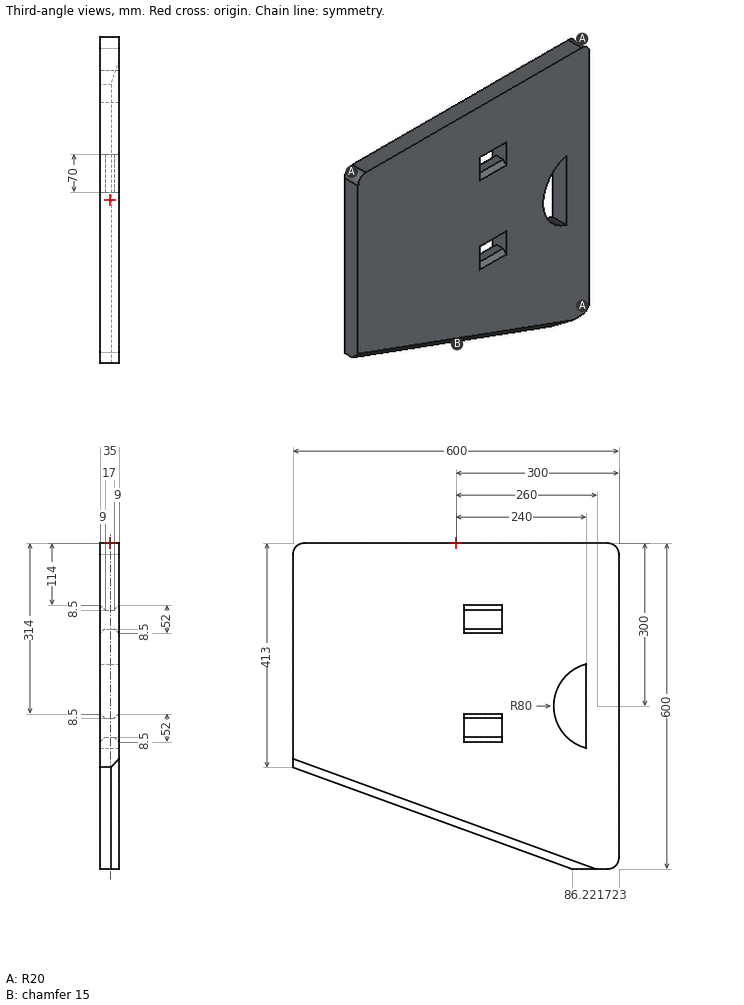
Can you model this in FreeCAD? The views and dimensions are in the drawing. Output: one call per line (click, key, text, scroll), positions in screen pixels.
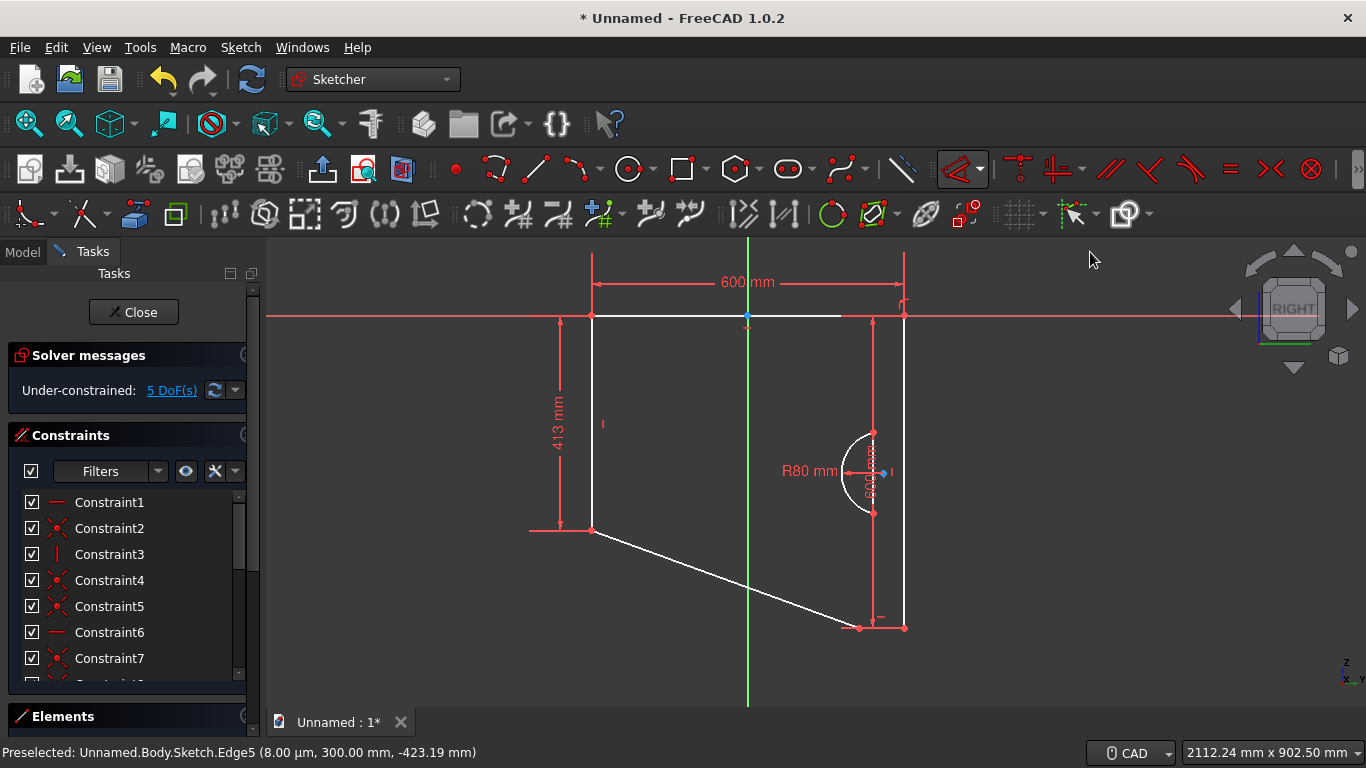
click(904, 316)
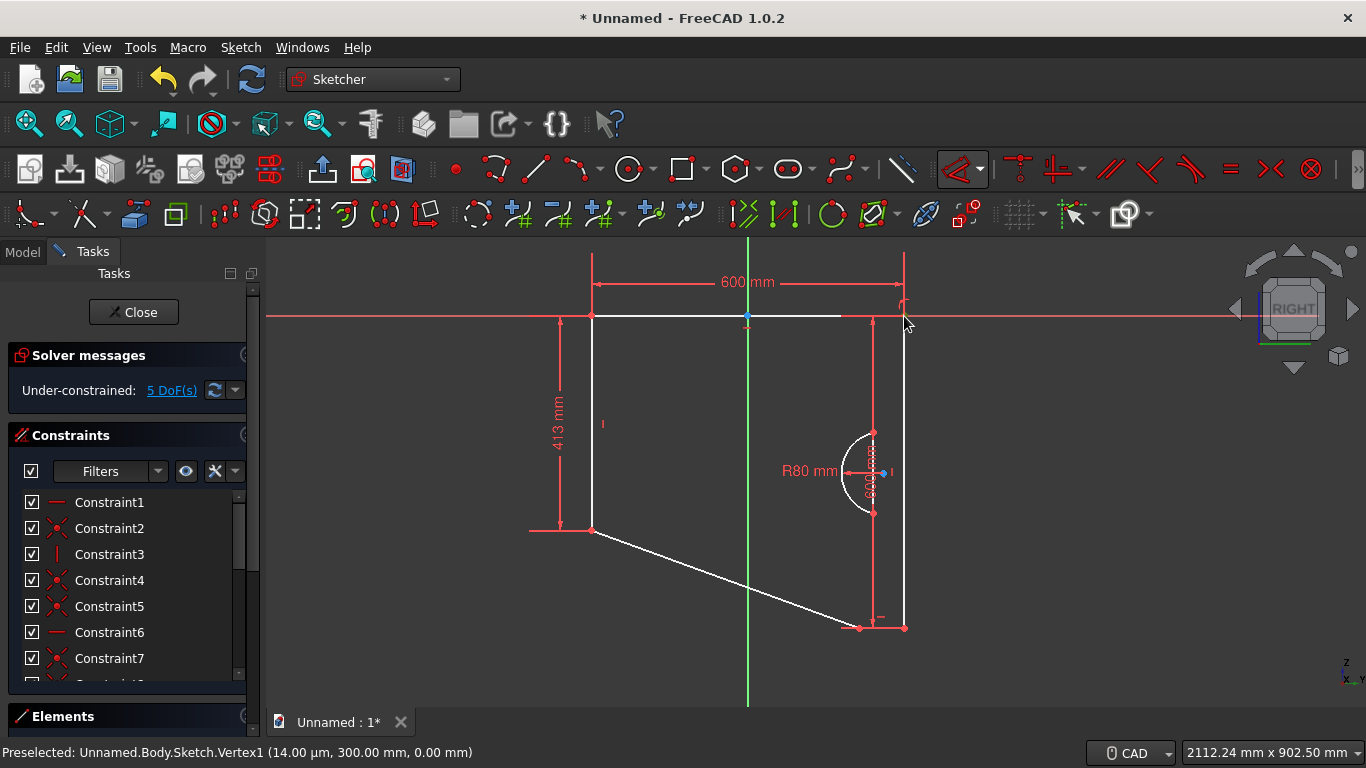
key(l)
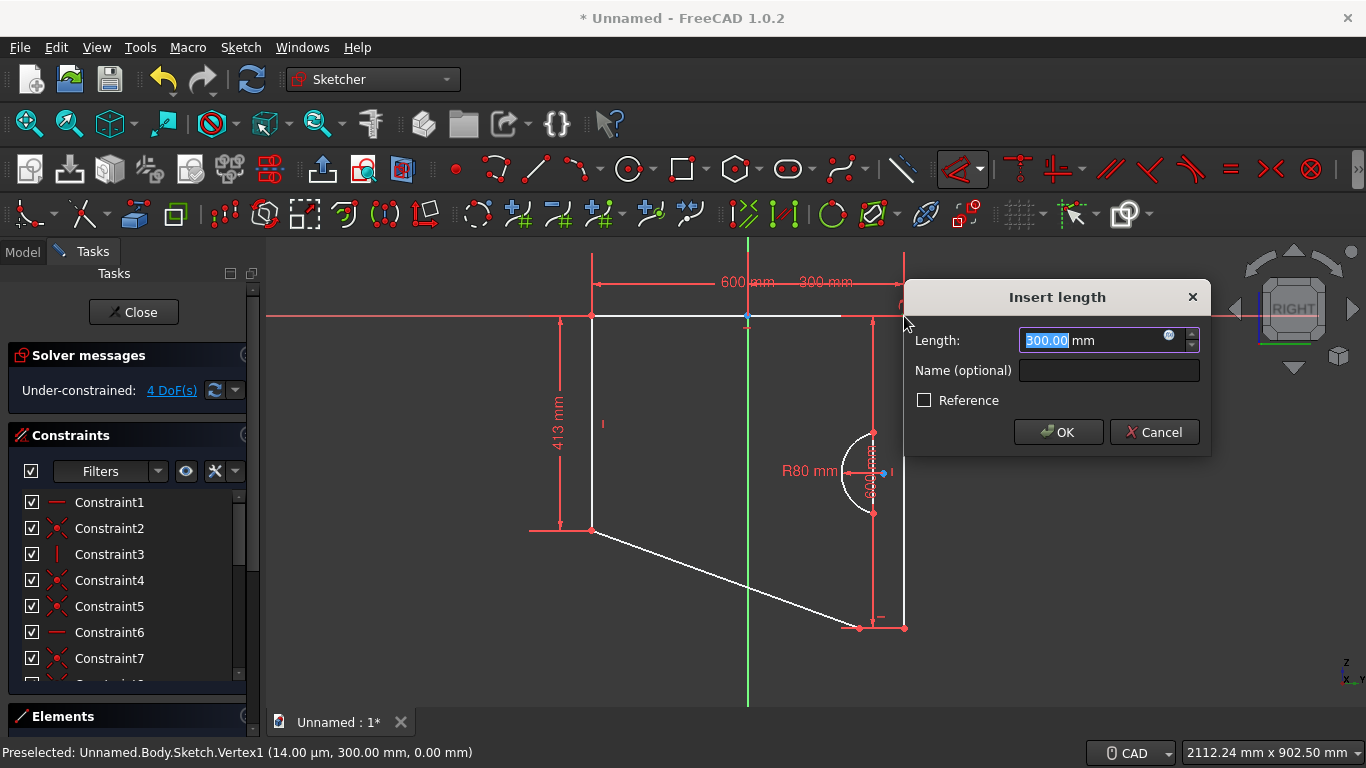
text(300)
key(Return)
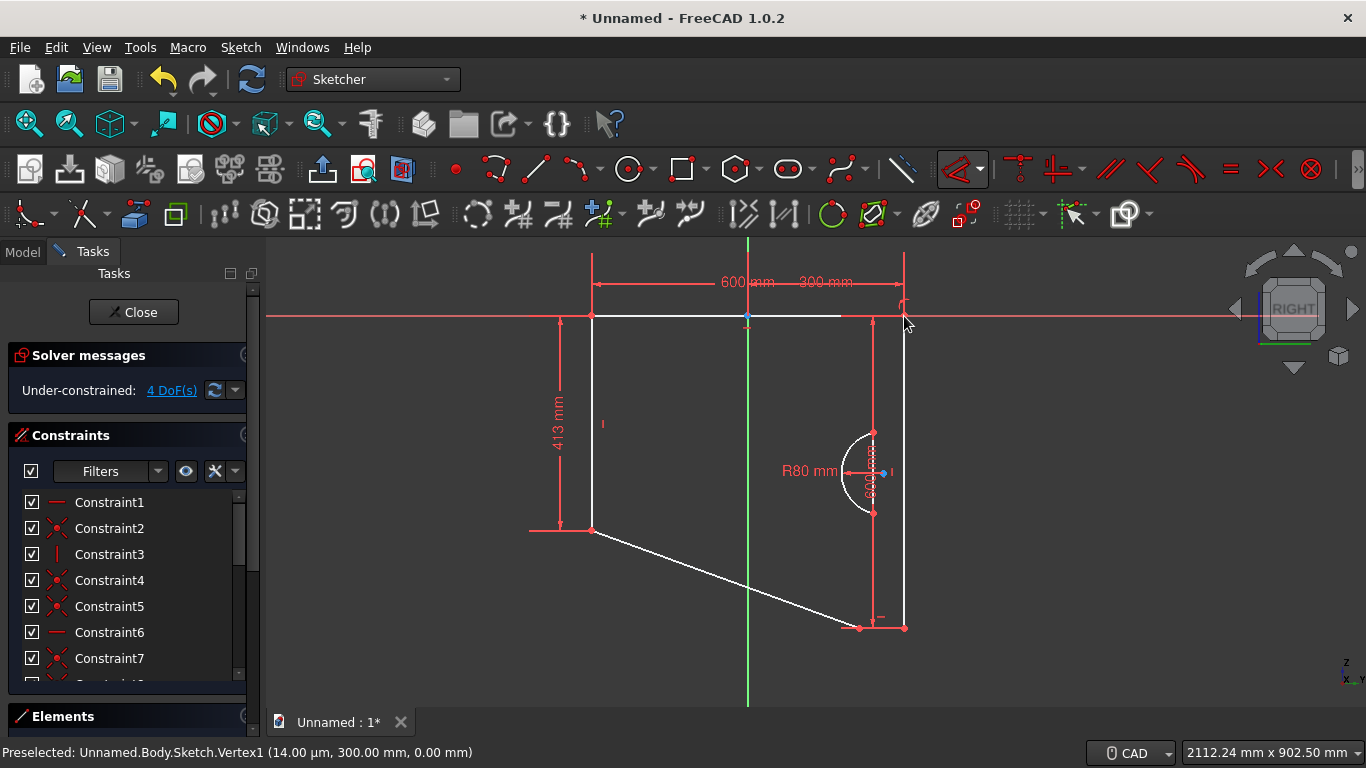
click(873, 433)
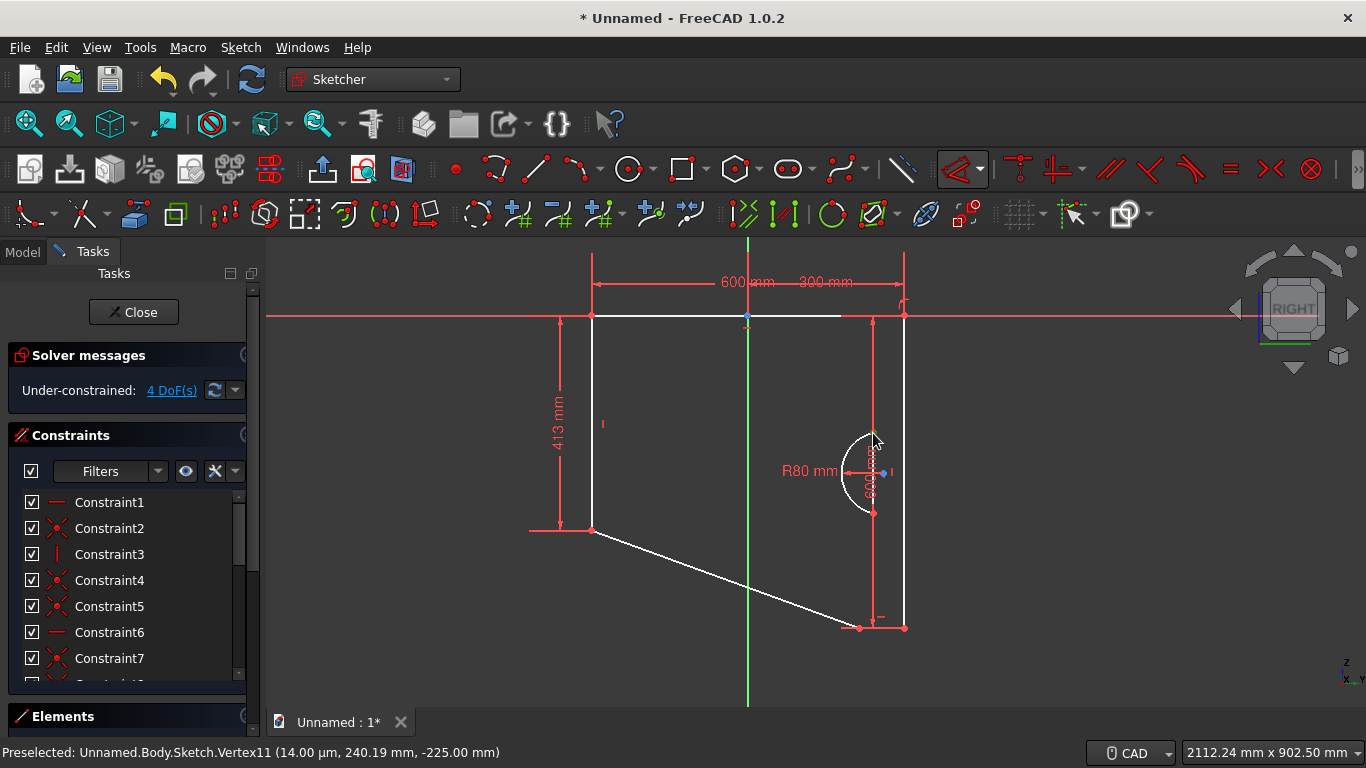
click(982, 170)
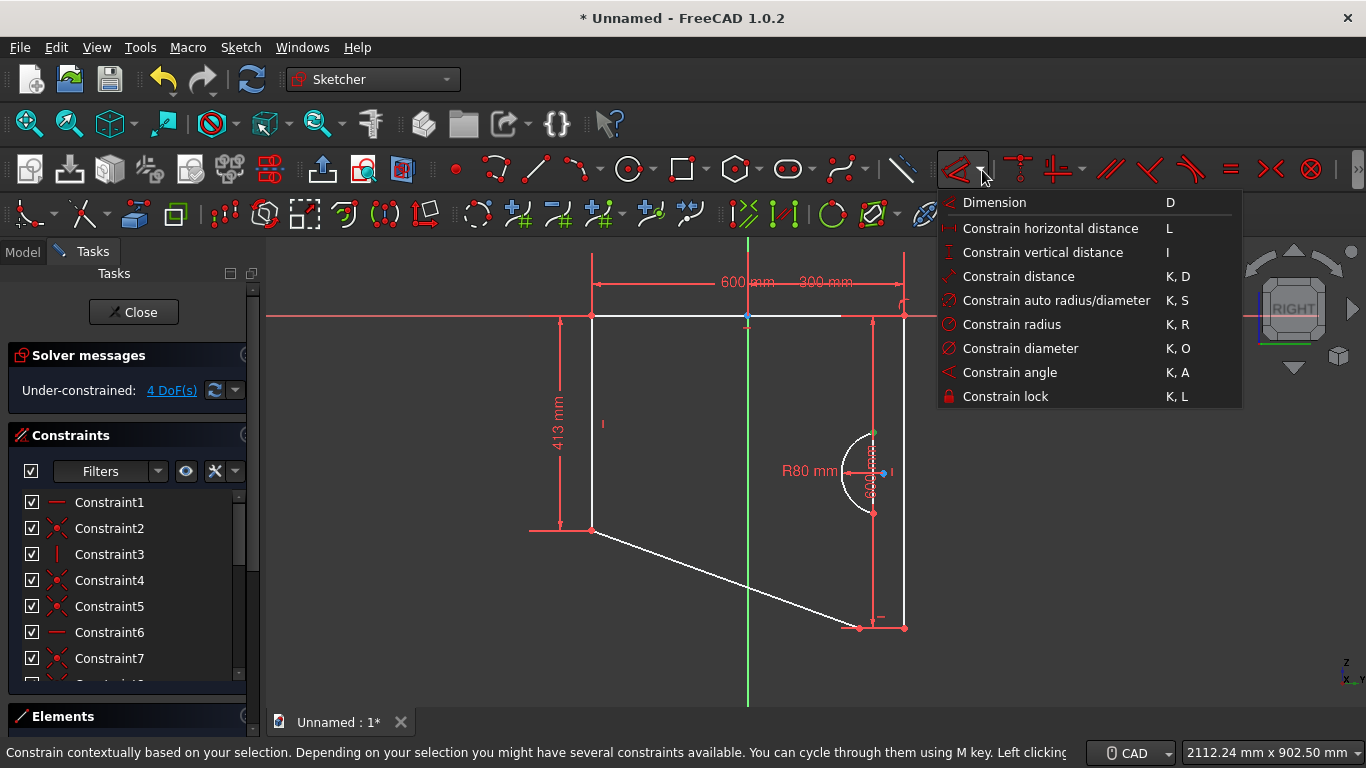
click(1090, 228)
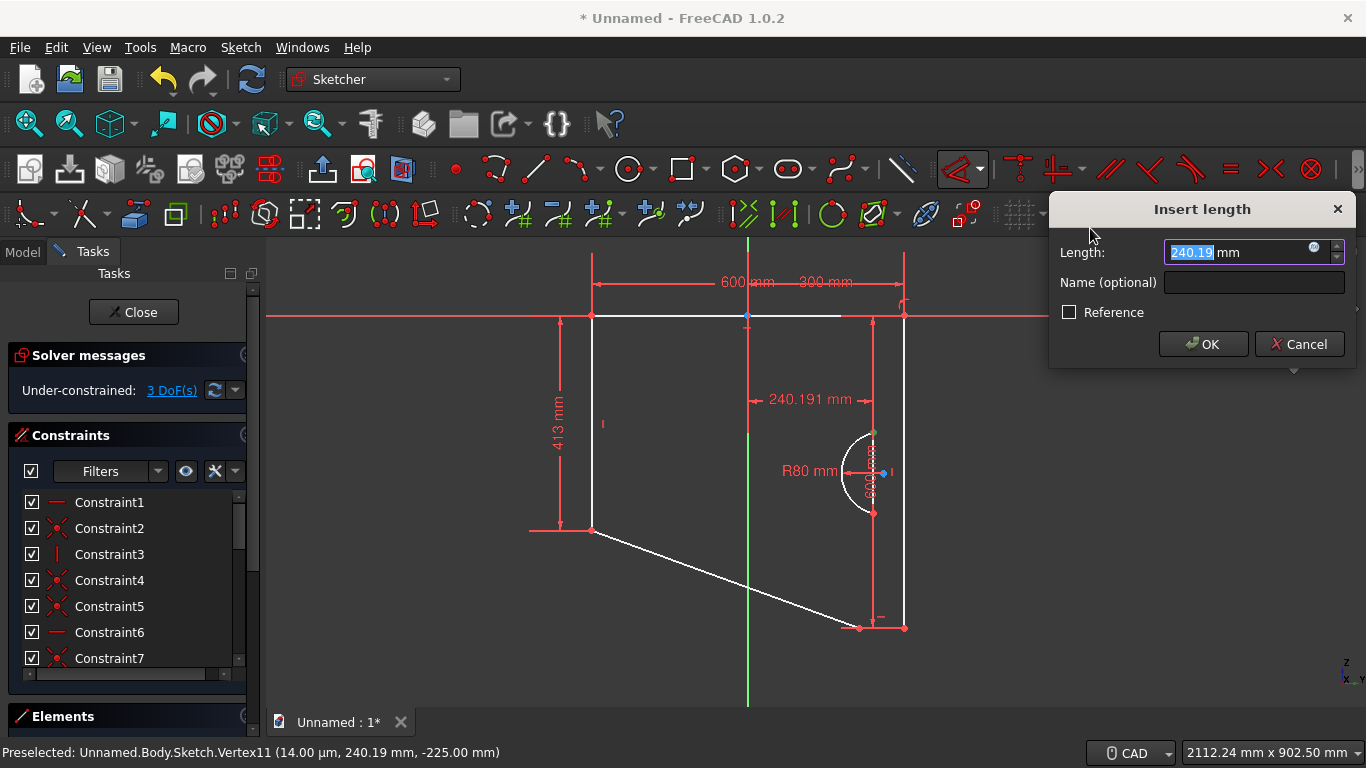
text(240)
key(Return)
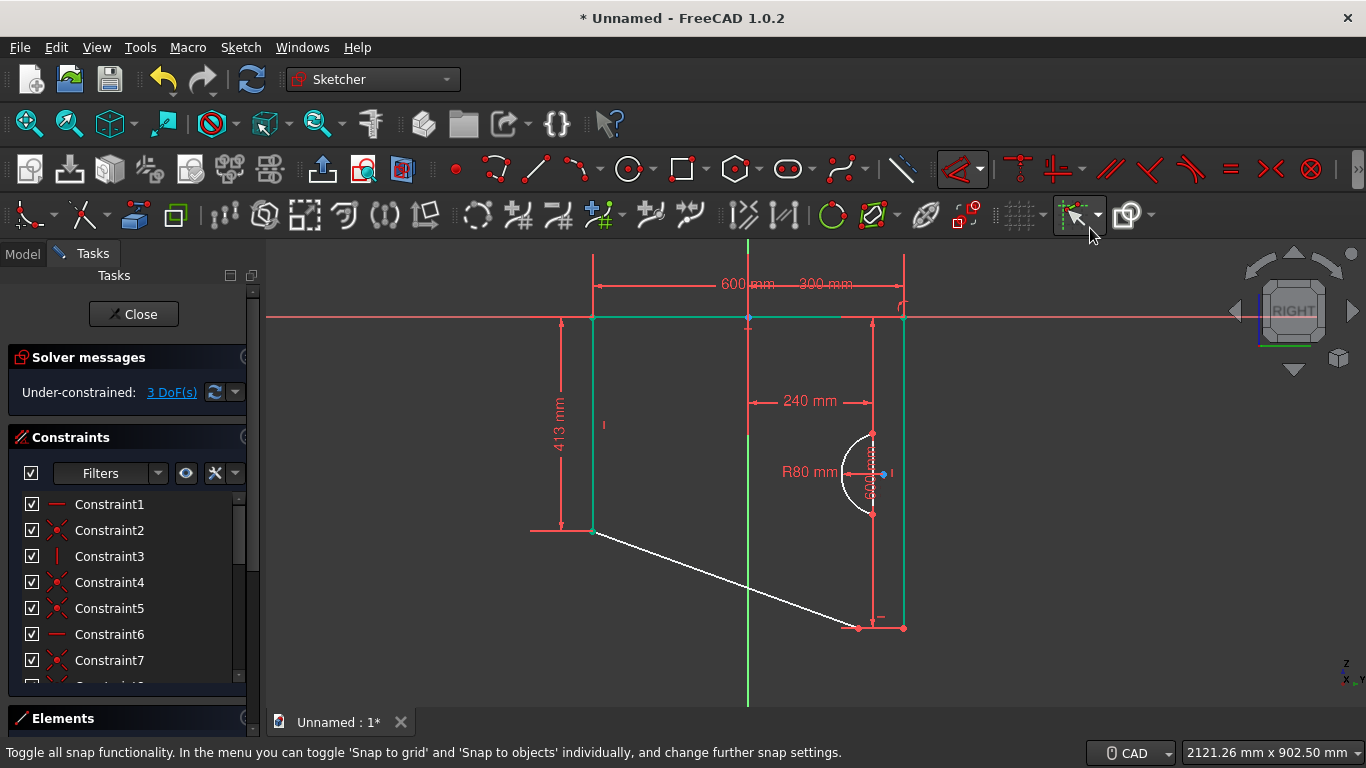
click(883, 474)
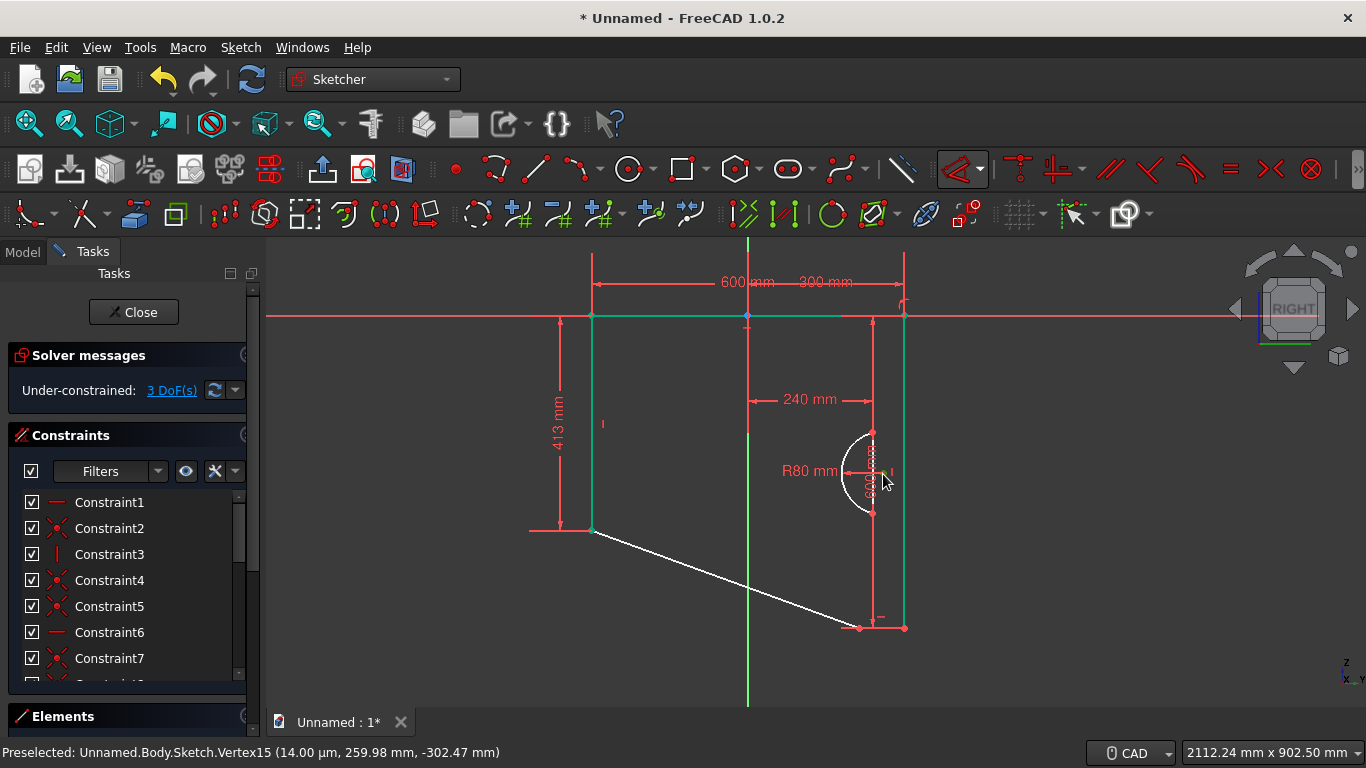
key(l)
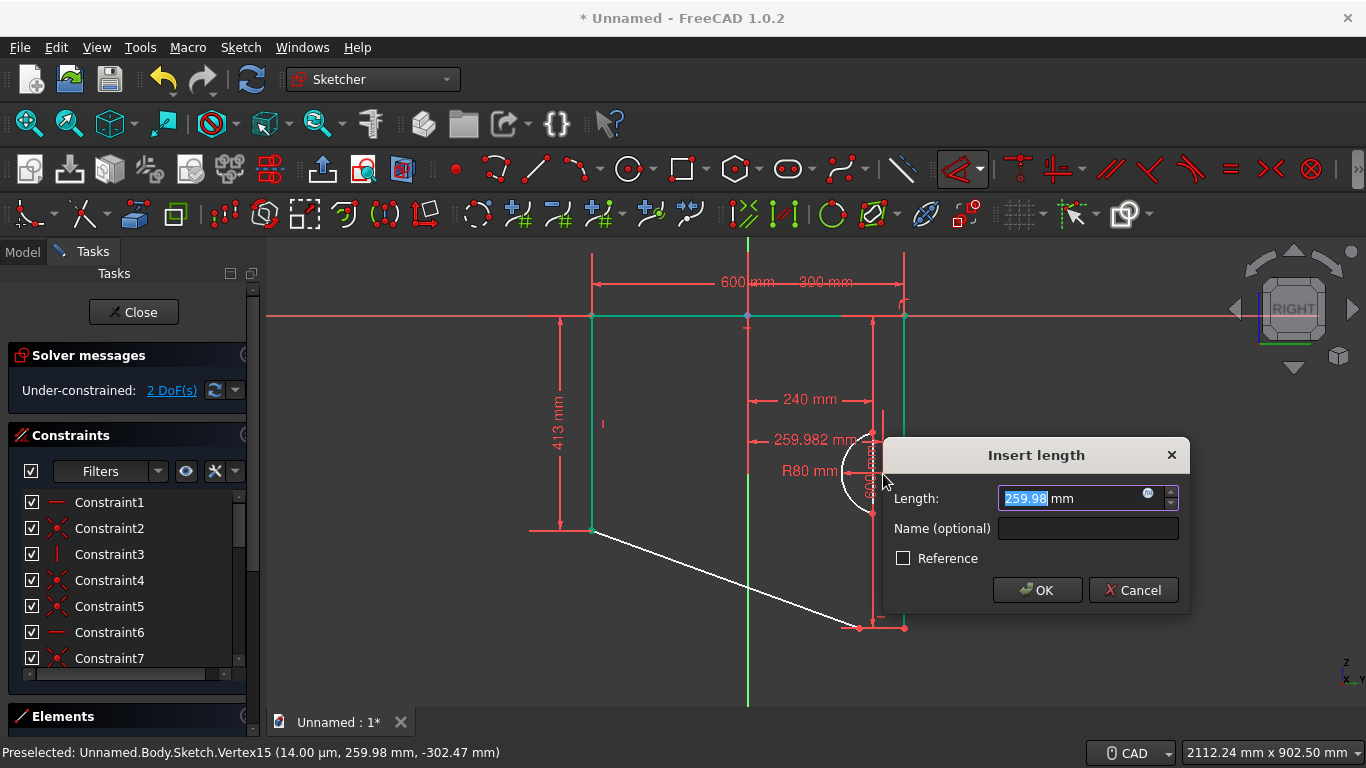
text(260)
key(Return)